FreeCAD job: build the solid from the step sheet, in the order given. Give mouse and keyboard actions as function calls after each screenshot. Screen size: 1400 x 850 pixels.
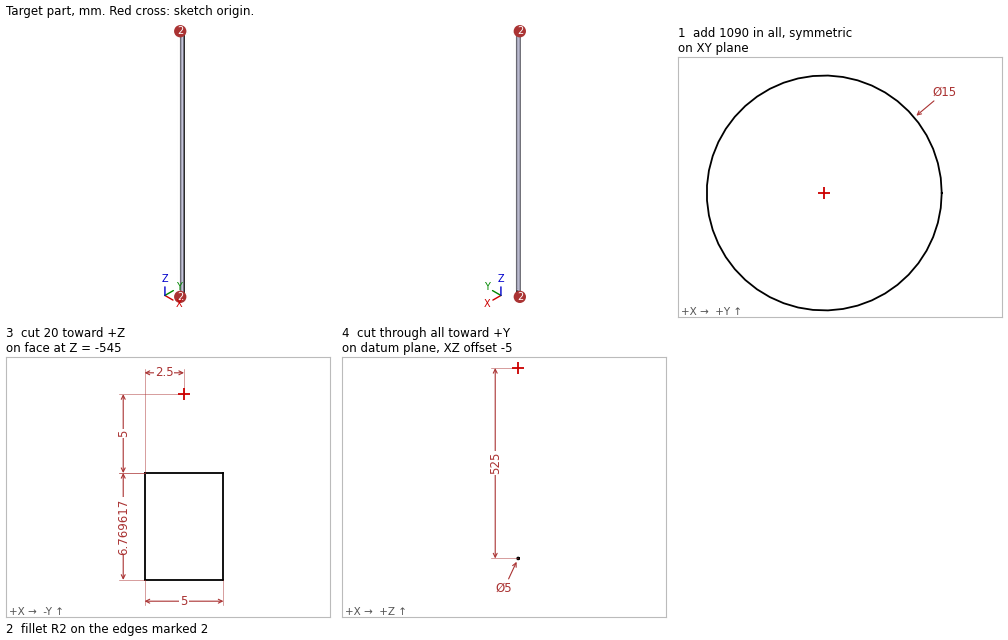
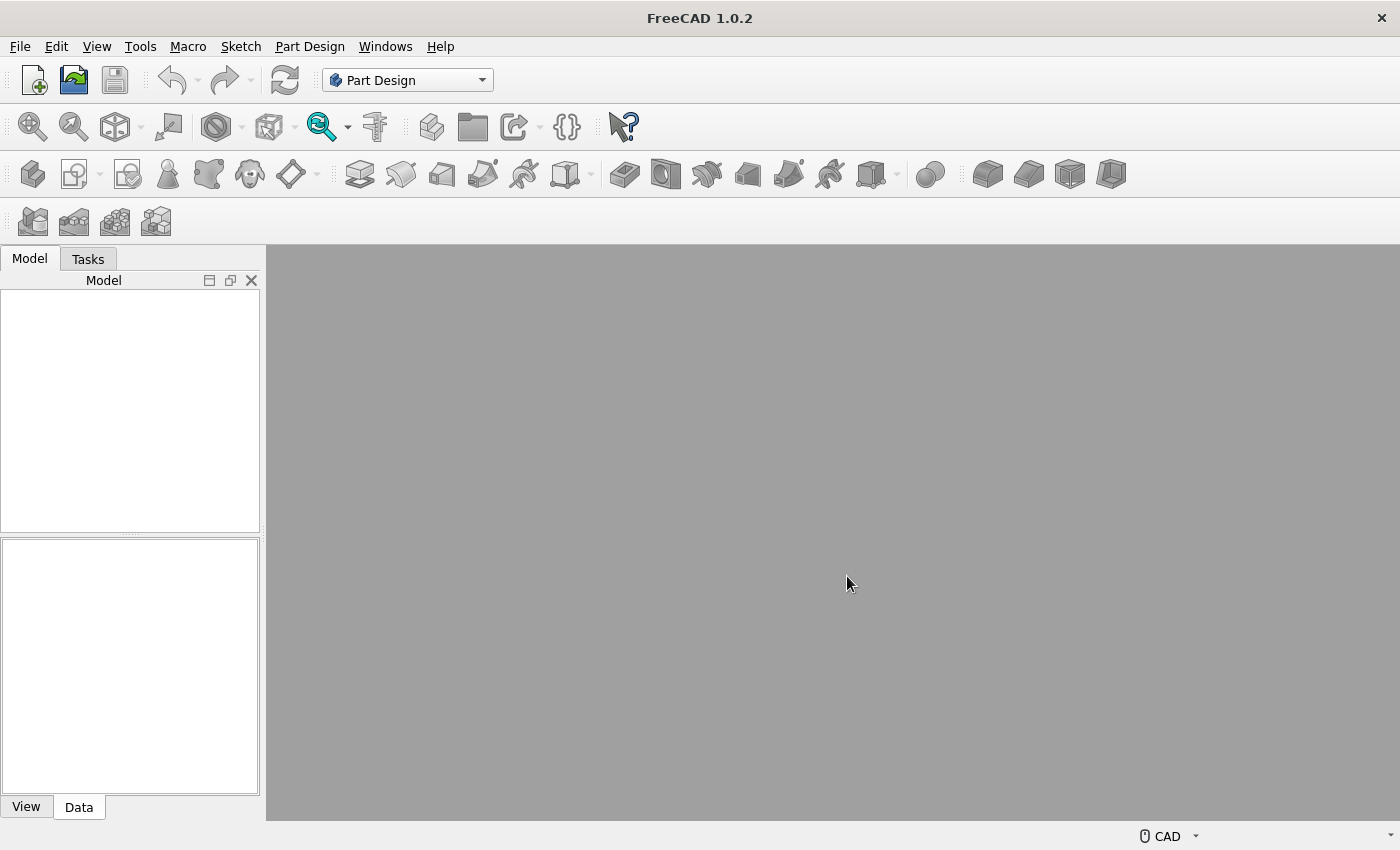
key(ctrl+n)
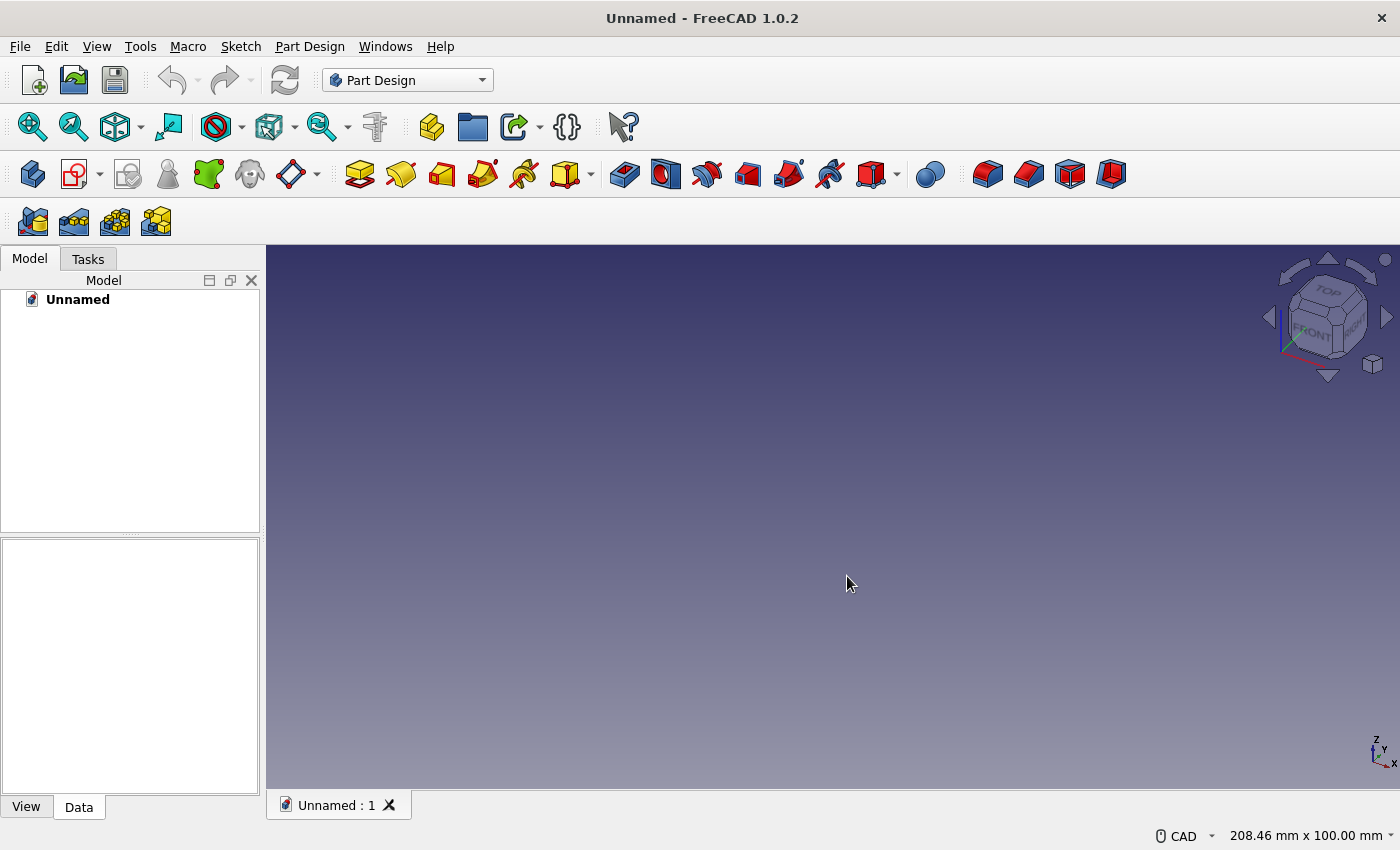
click(74, 174)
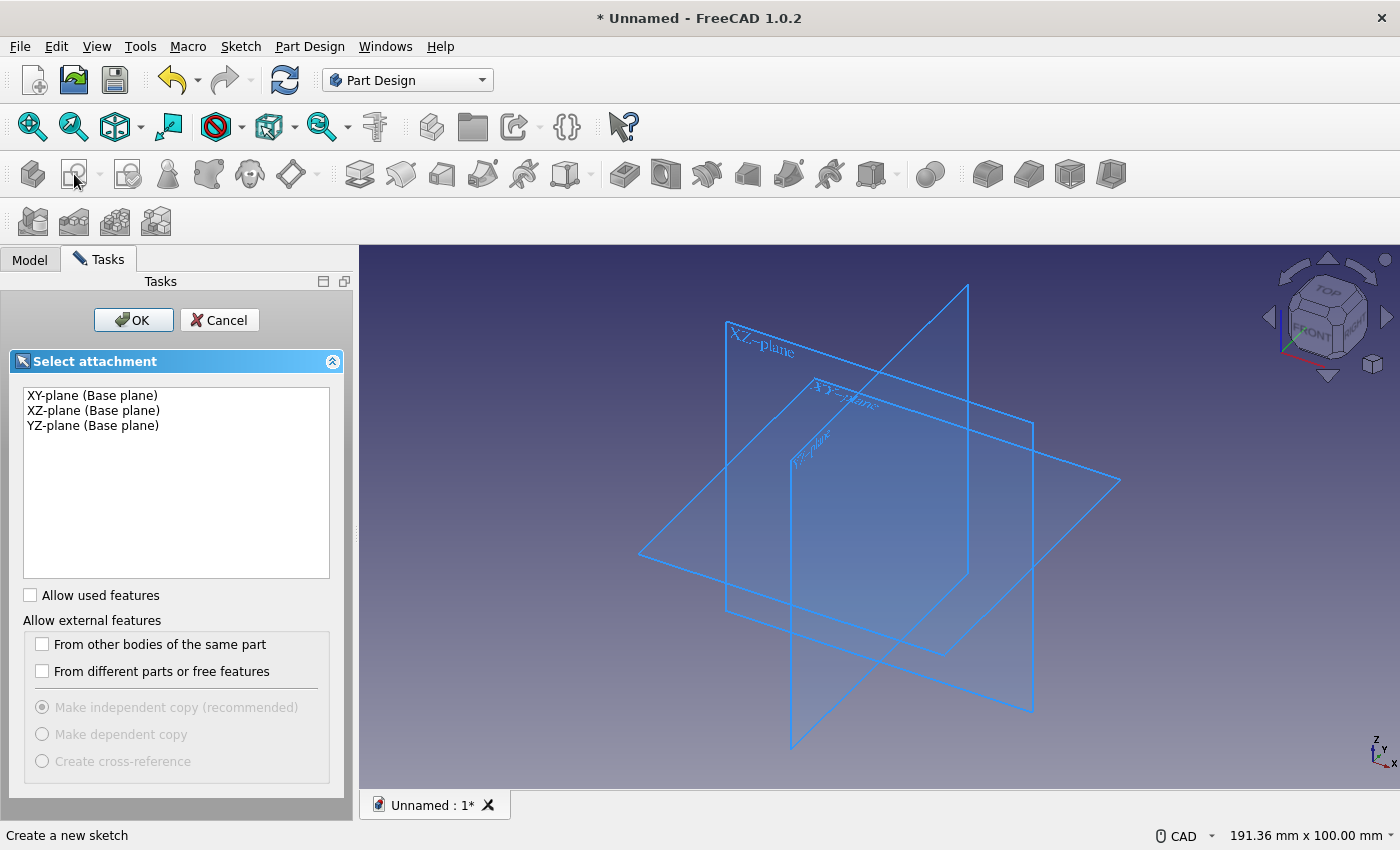
click(84, 396)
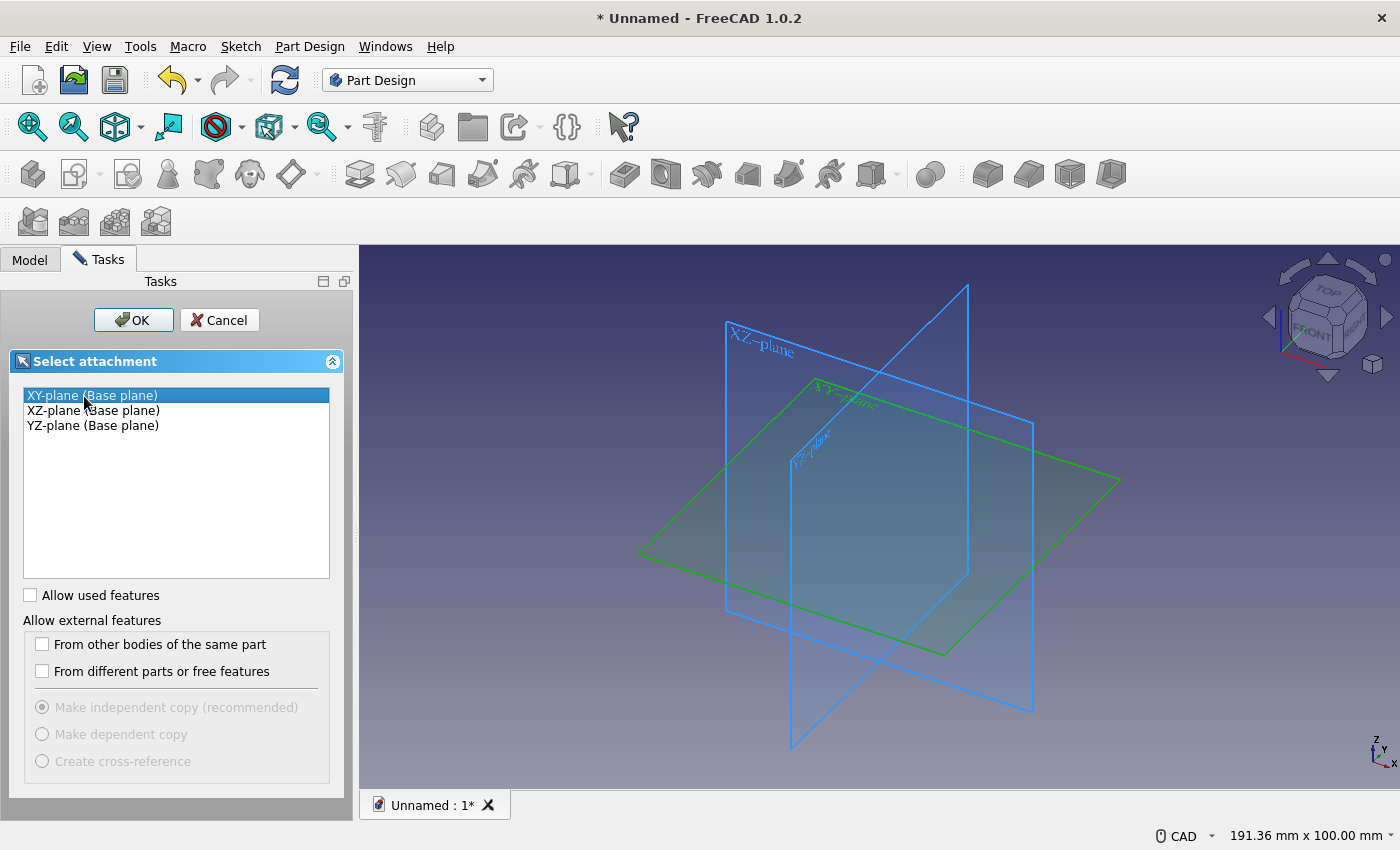
click(134, 320)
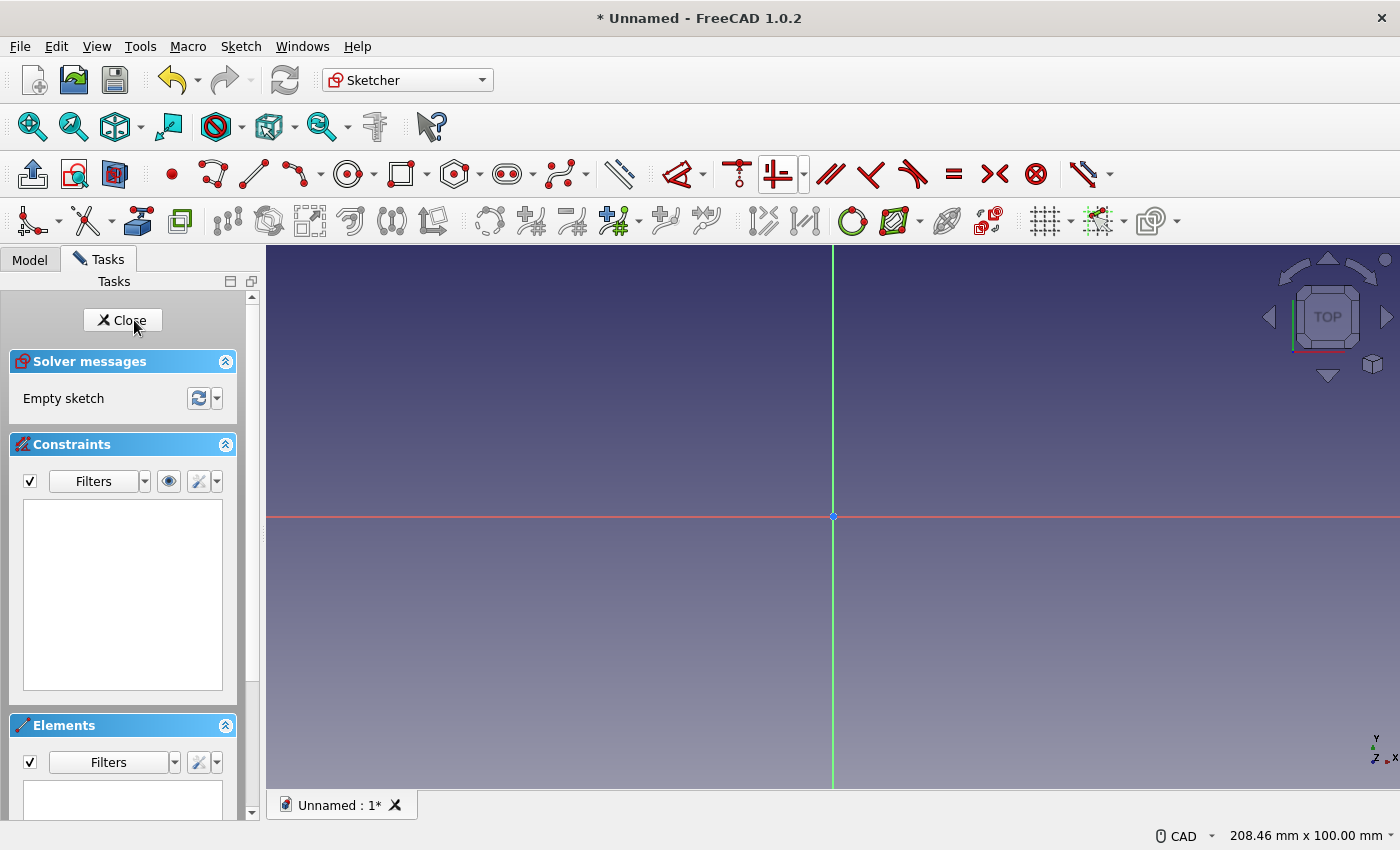
scroll(855, 517, up, 7)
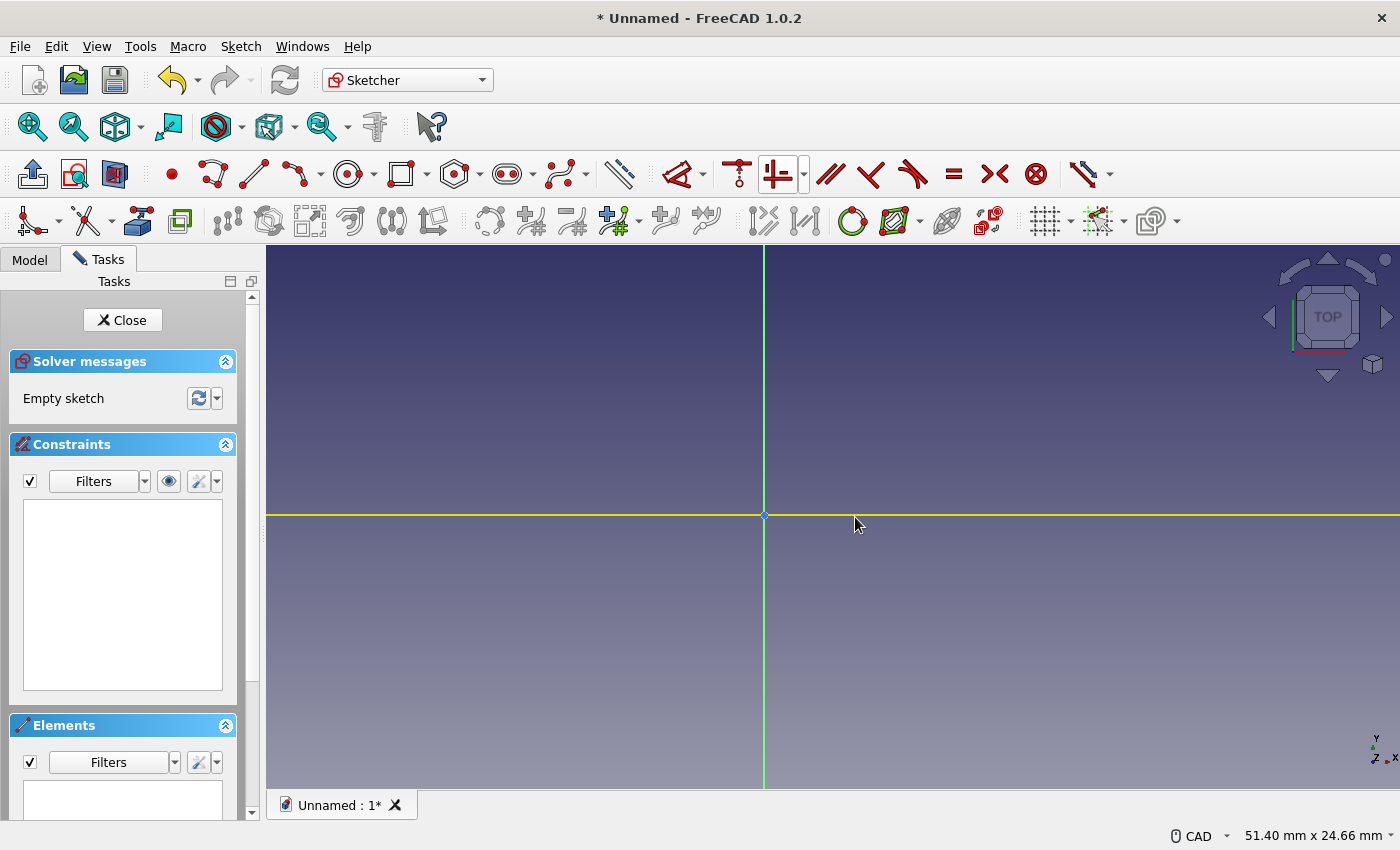
click(348, 174)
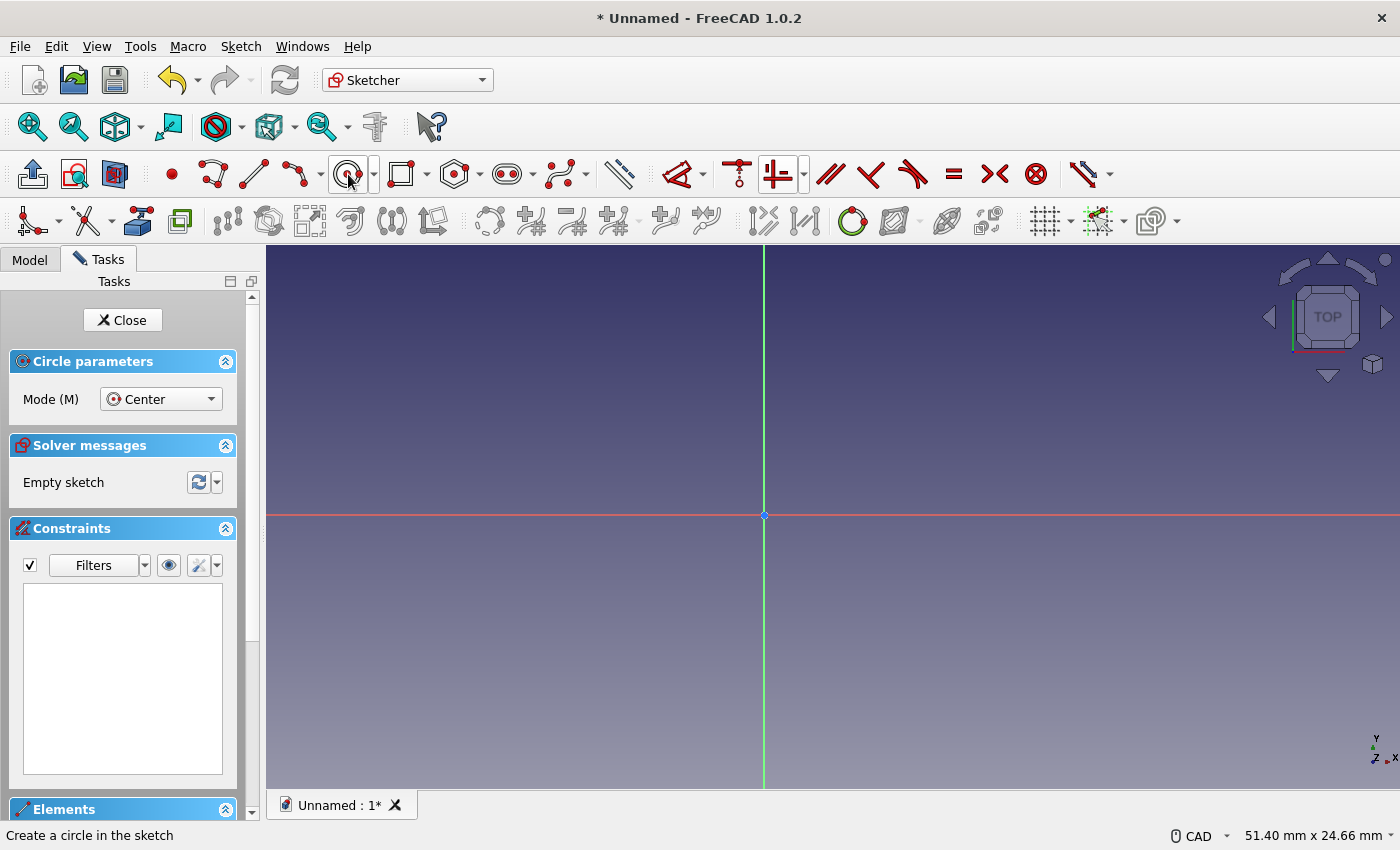
click(764, 515)
click(881, 398)
key(Escape)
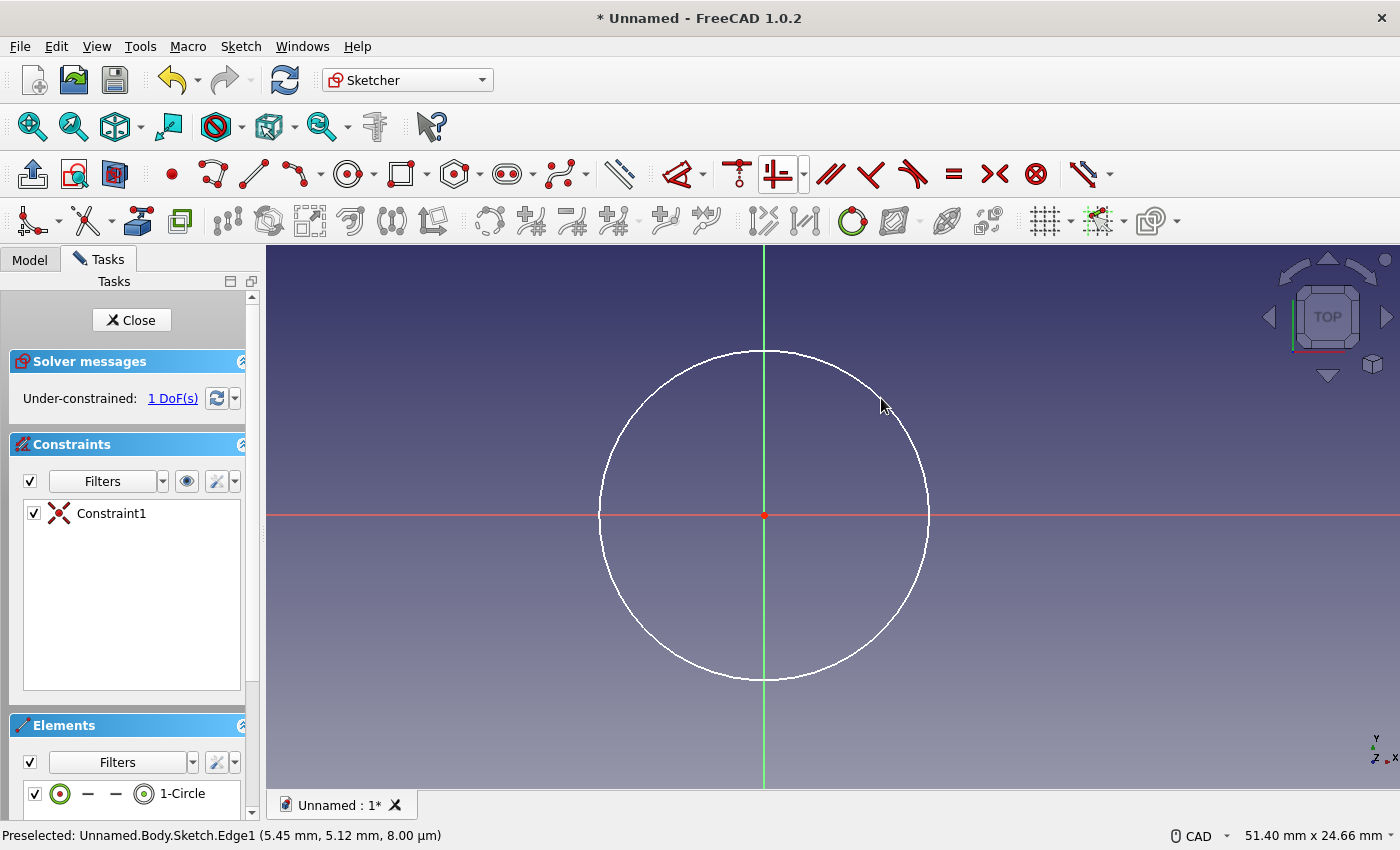
key(d)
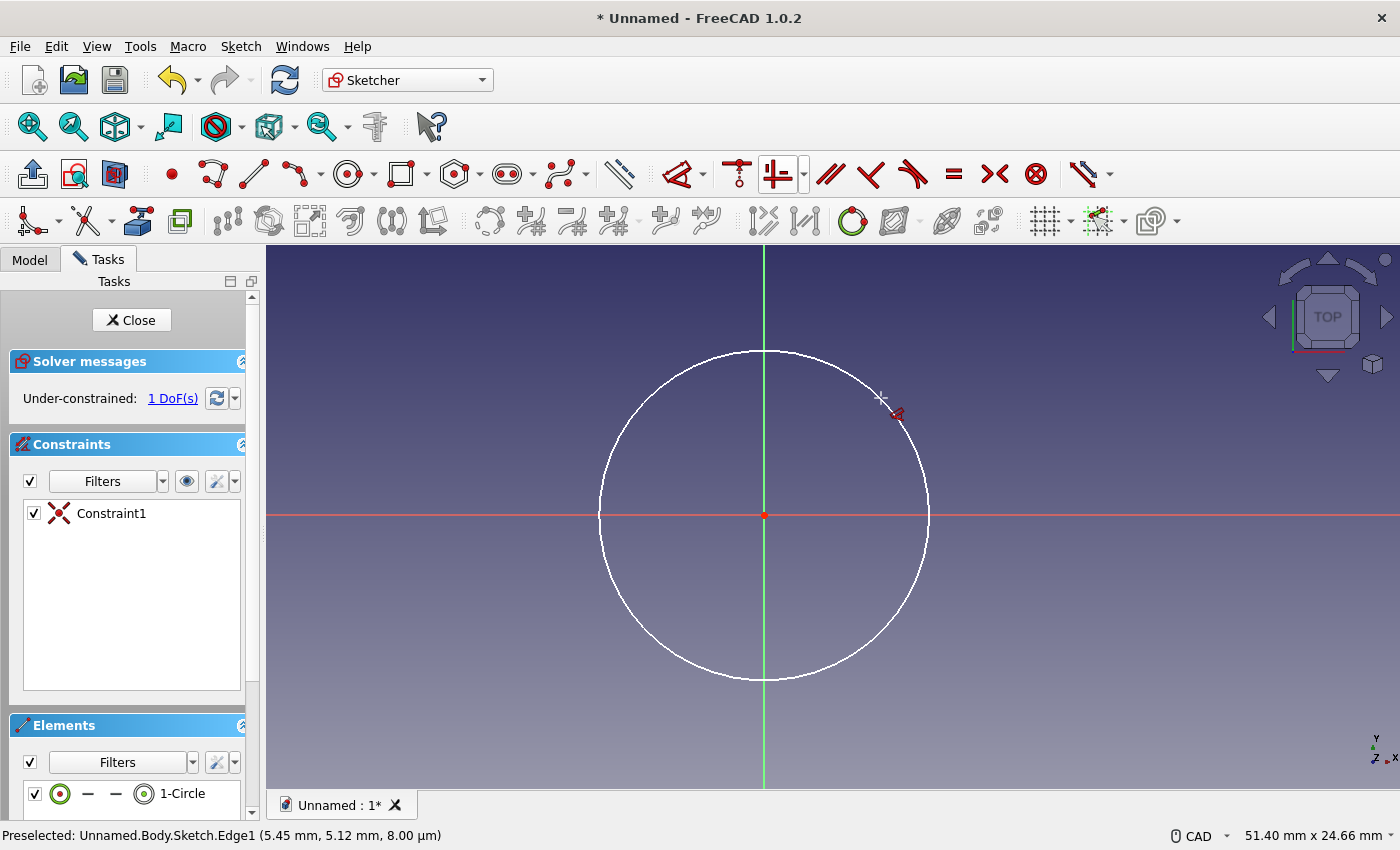
click(880, 398)
click(902, 375)